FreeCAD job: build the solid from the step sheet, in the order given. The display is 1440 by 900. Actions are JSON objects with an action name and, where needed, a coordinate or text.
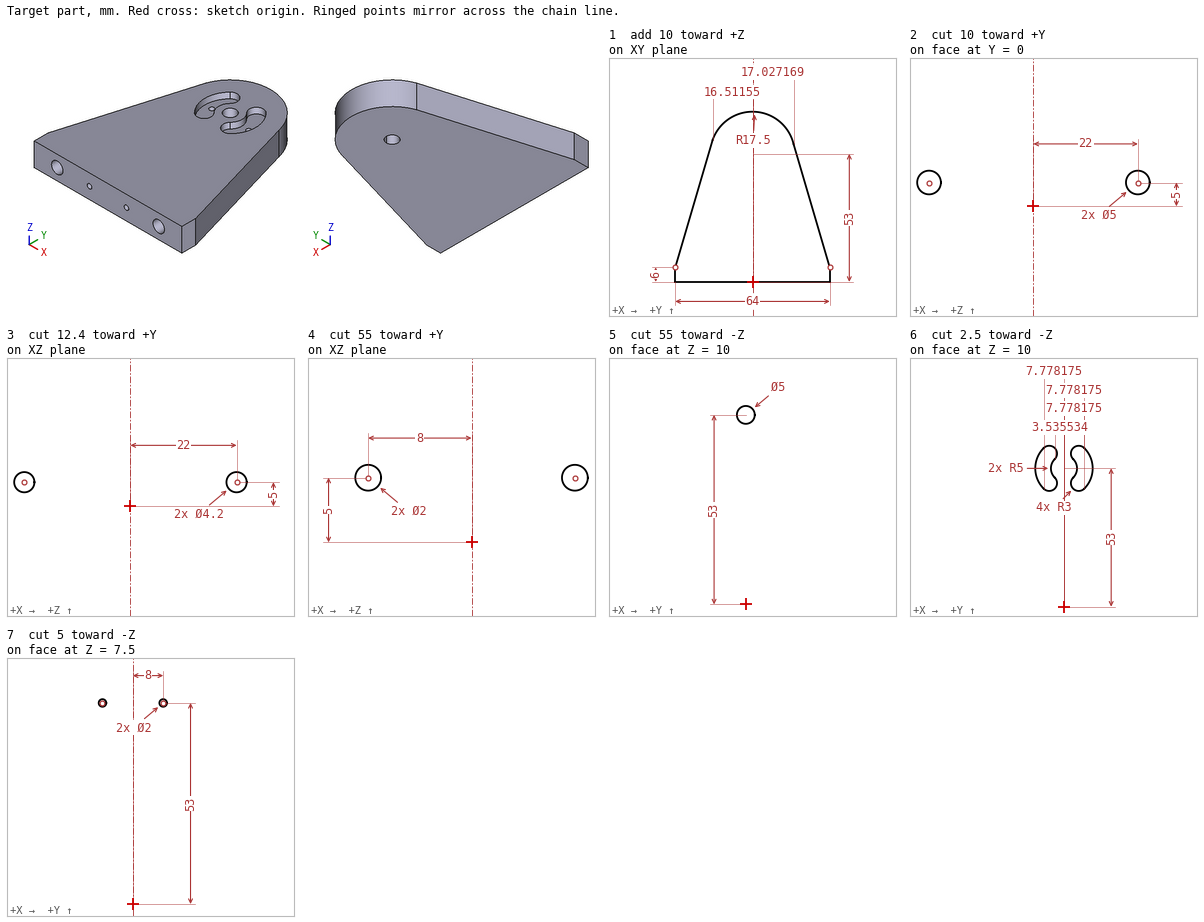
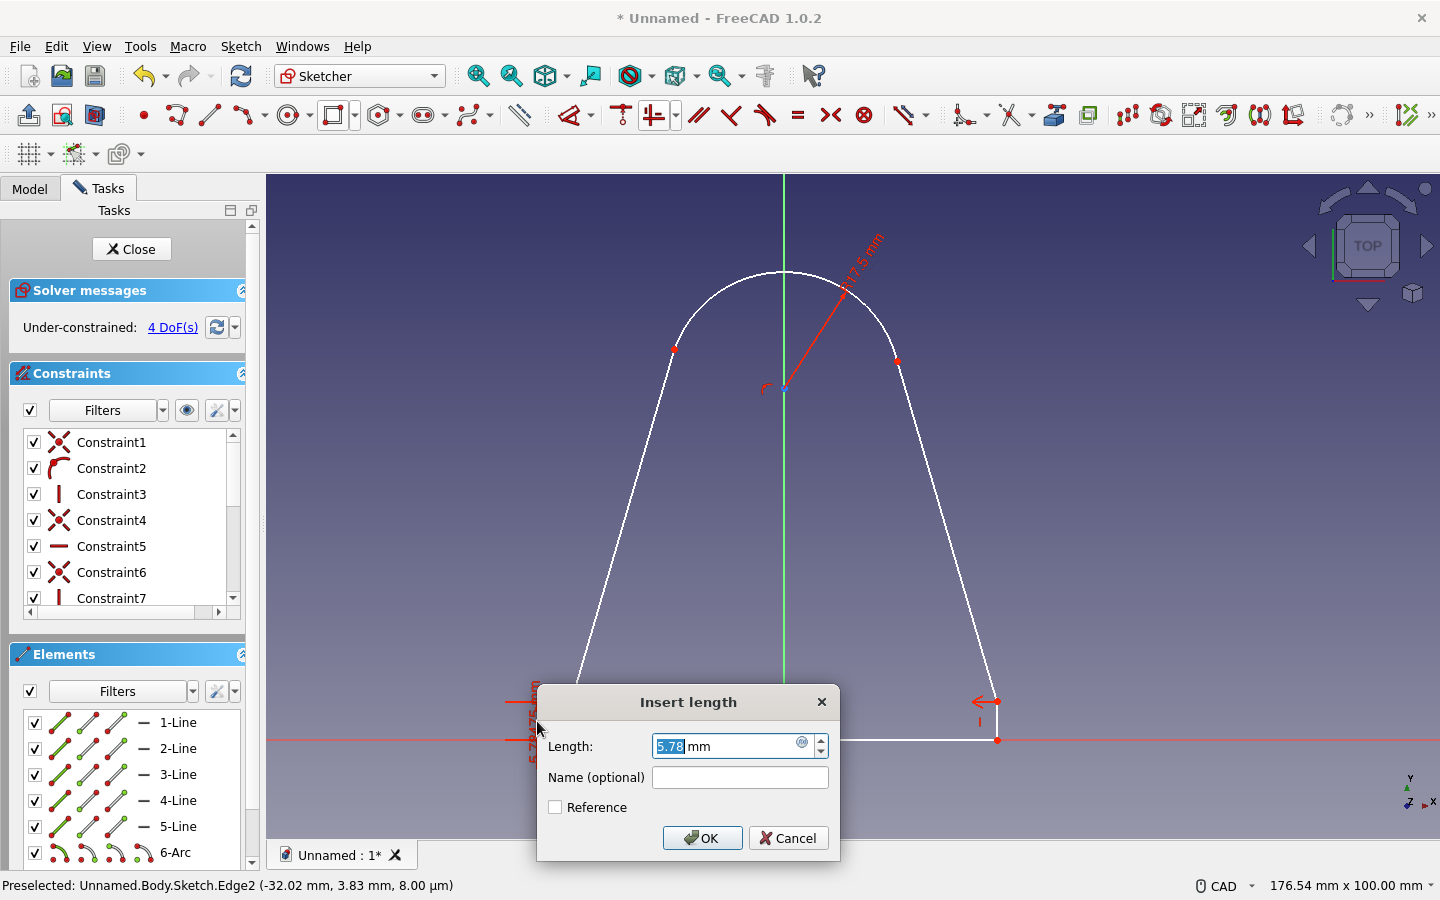
{"action": "type", "text": "6"}
{"action": "key", "text": "Return"}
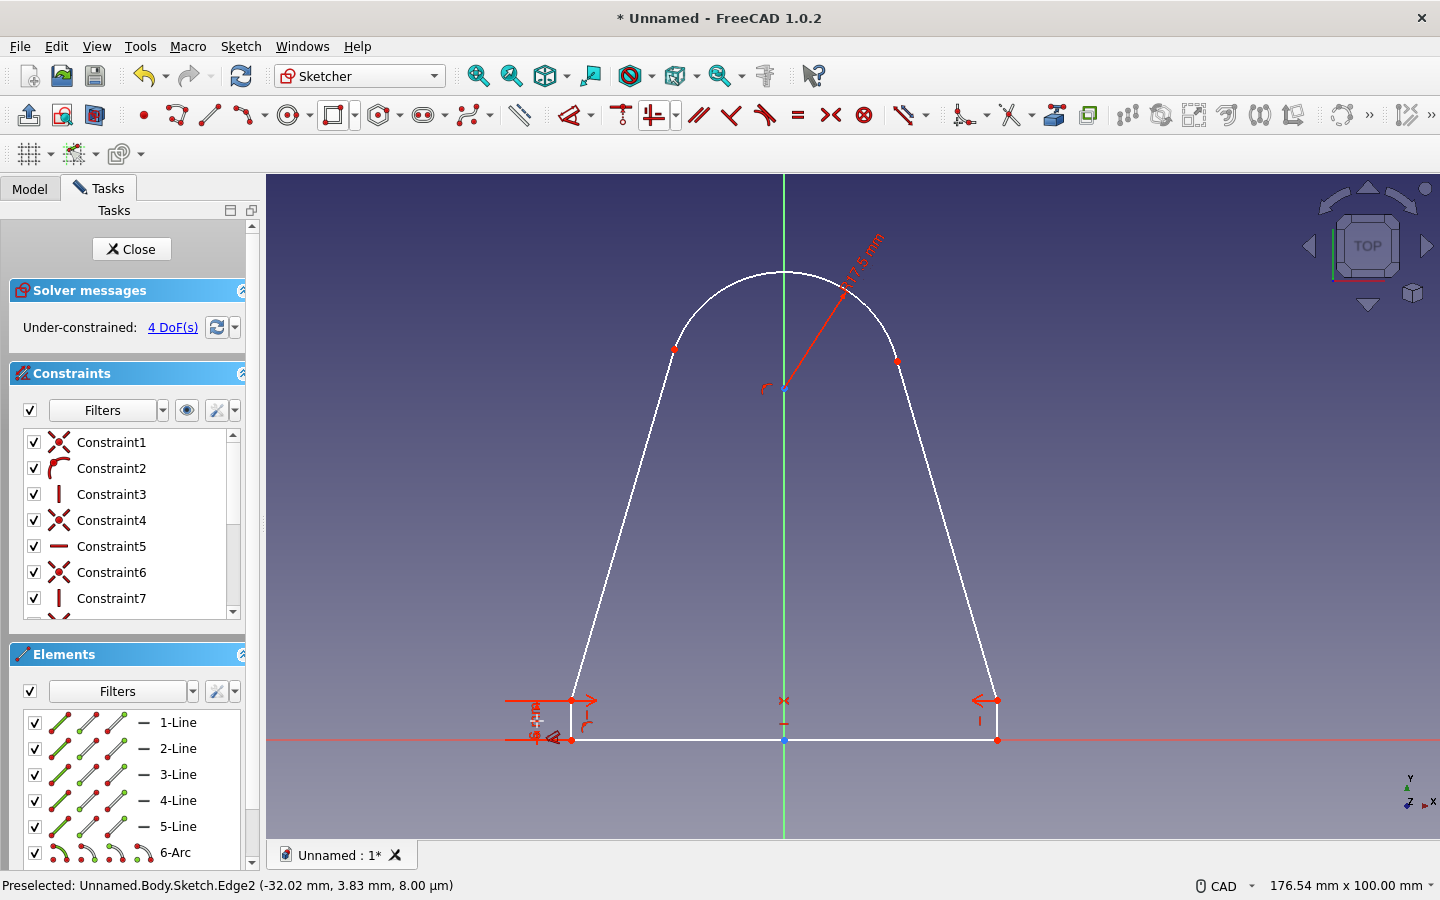
{"action": "left_click", "coordinate": [699, 740]}
{"action": "left_click", "coordinate": [686, 774]}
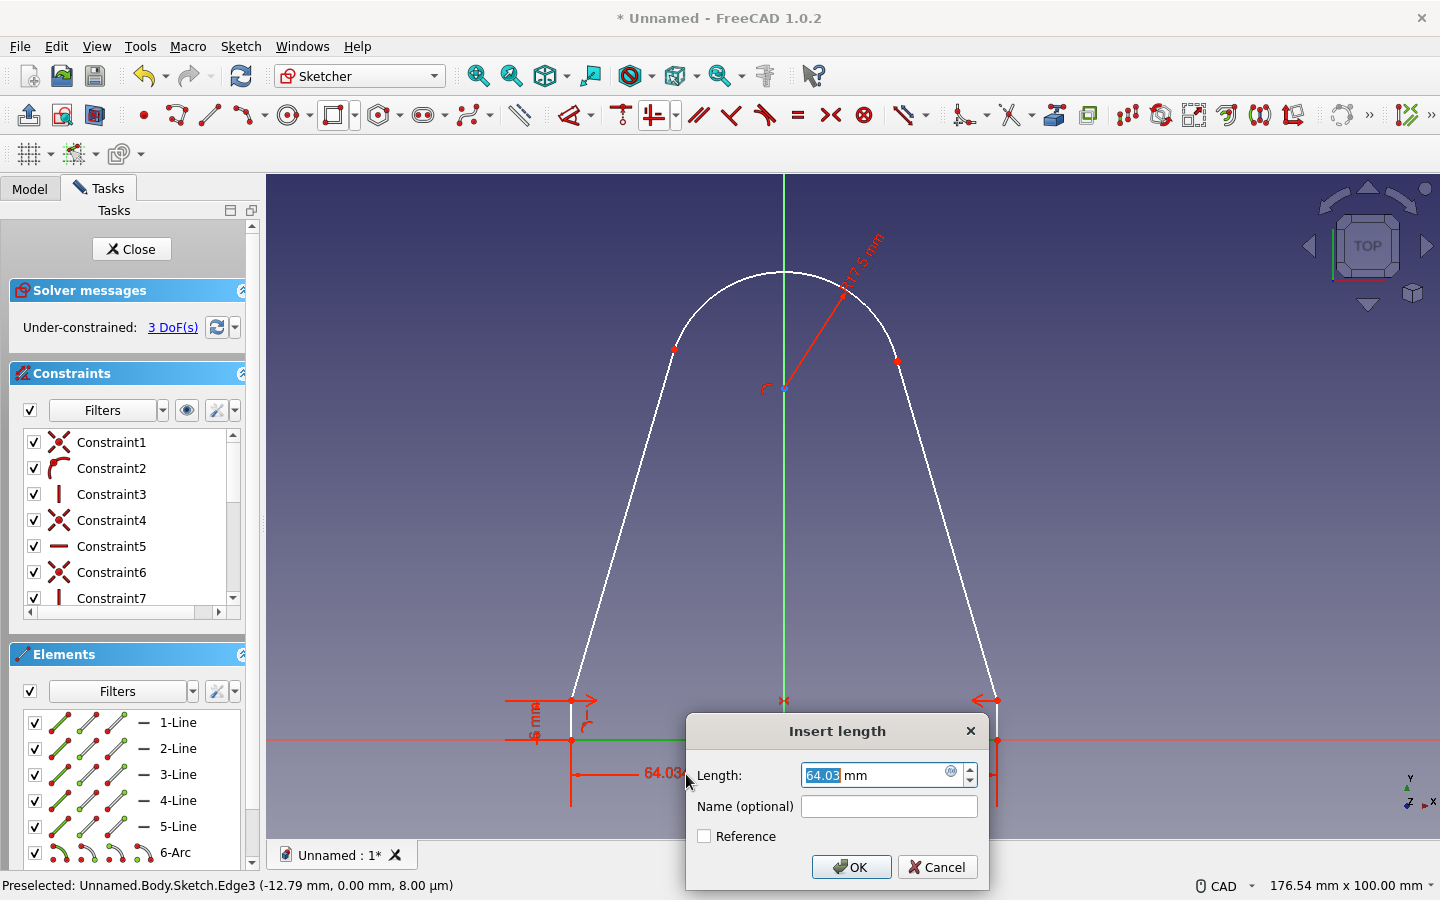
{"action": "type", "text": "64"}
{"action": "key", "text": "Return"}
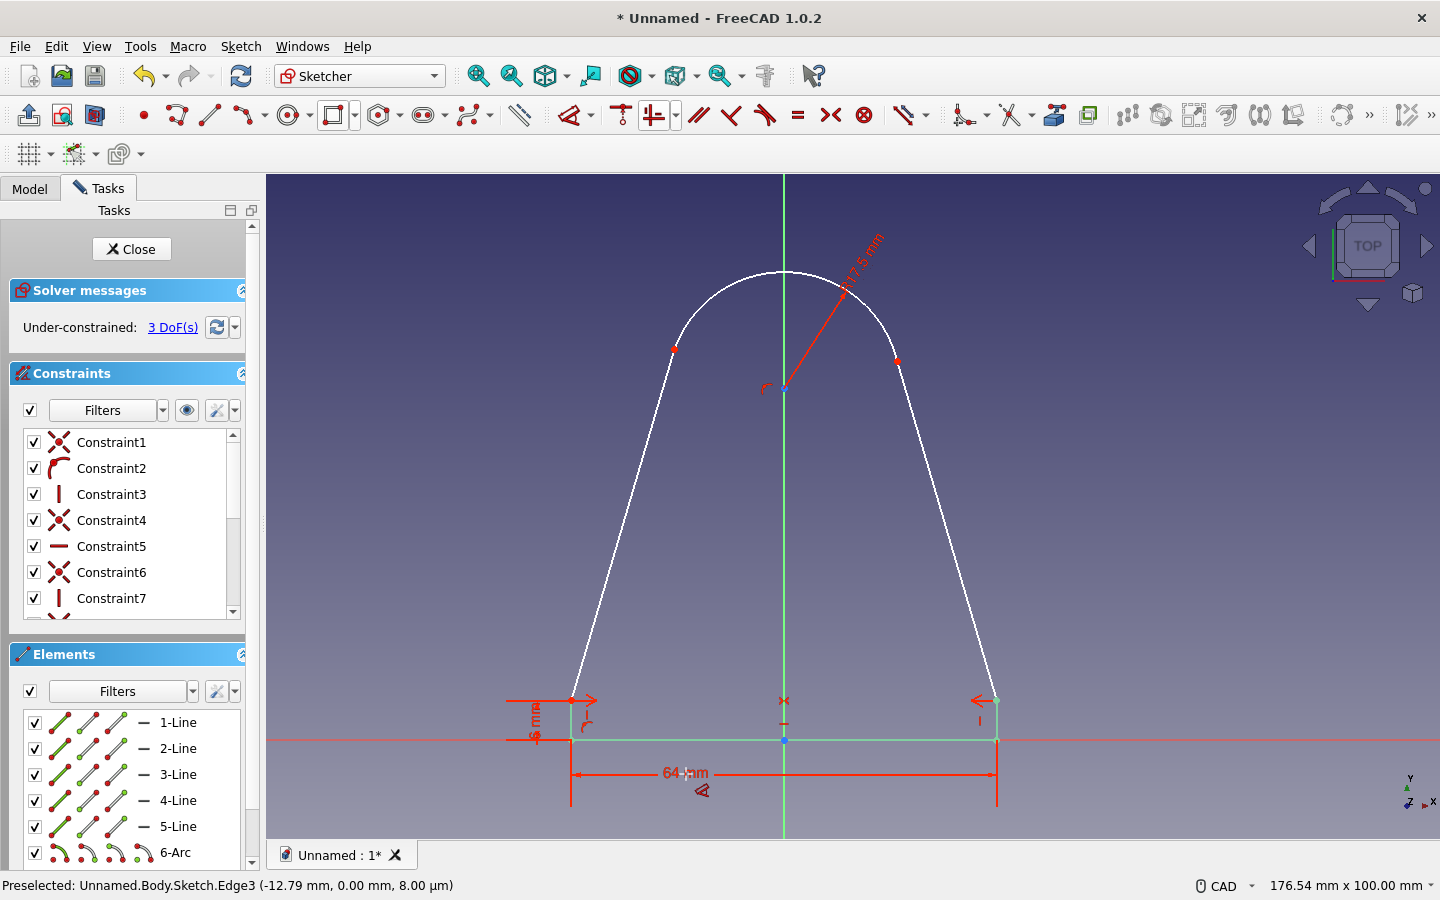
{"action": "left_click", "coordinate": [784, 389]}
{"action": "left_click", "coordinate": [818, 564]}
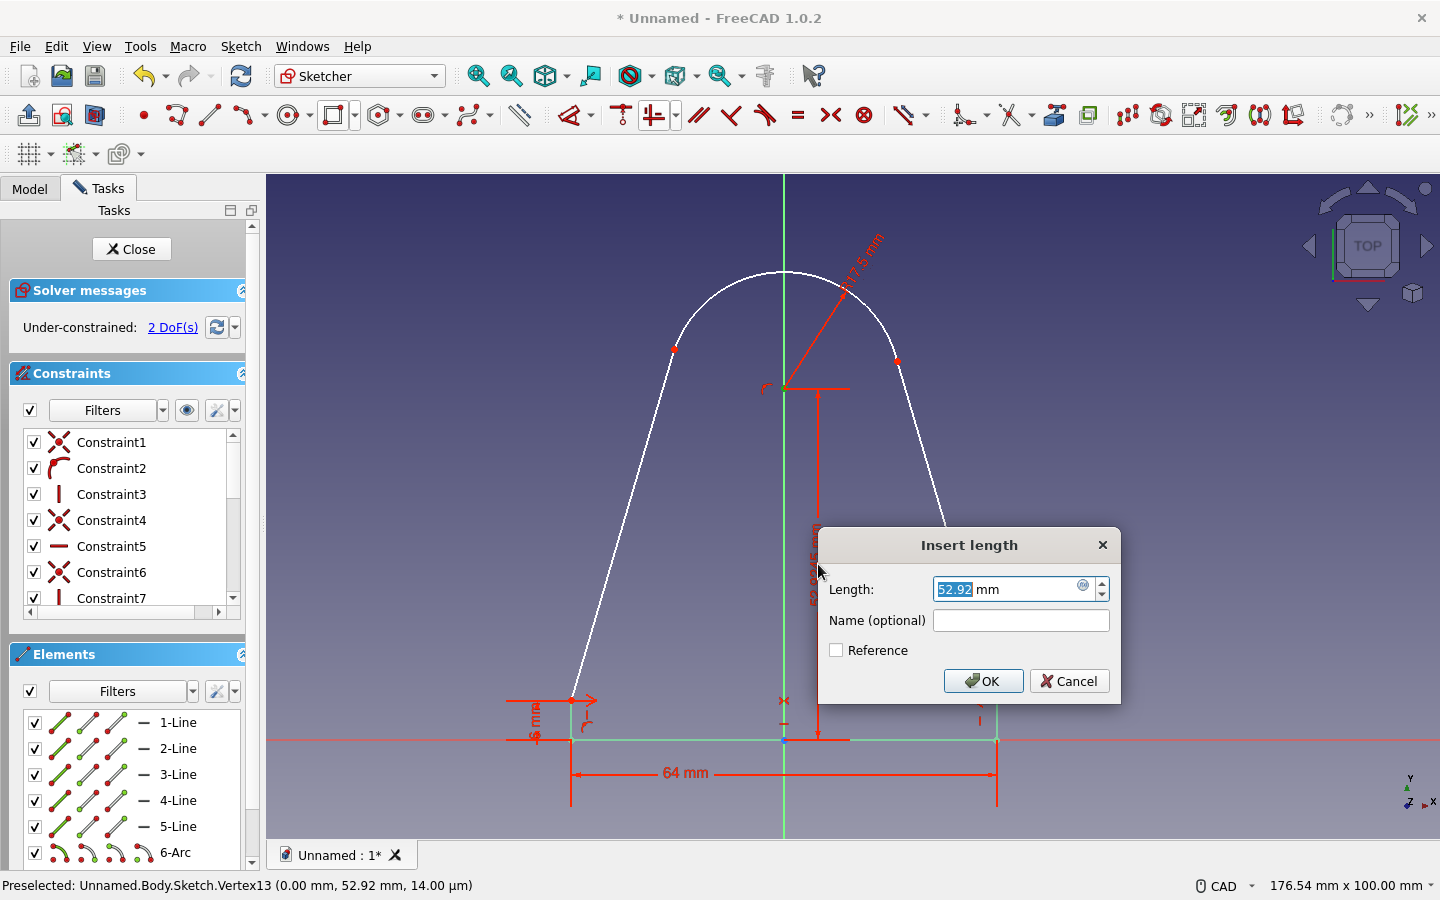
{"action": "type", "text": "53"}
{"action": "key", "text": "Return"}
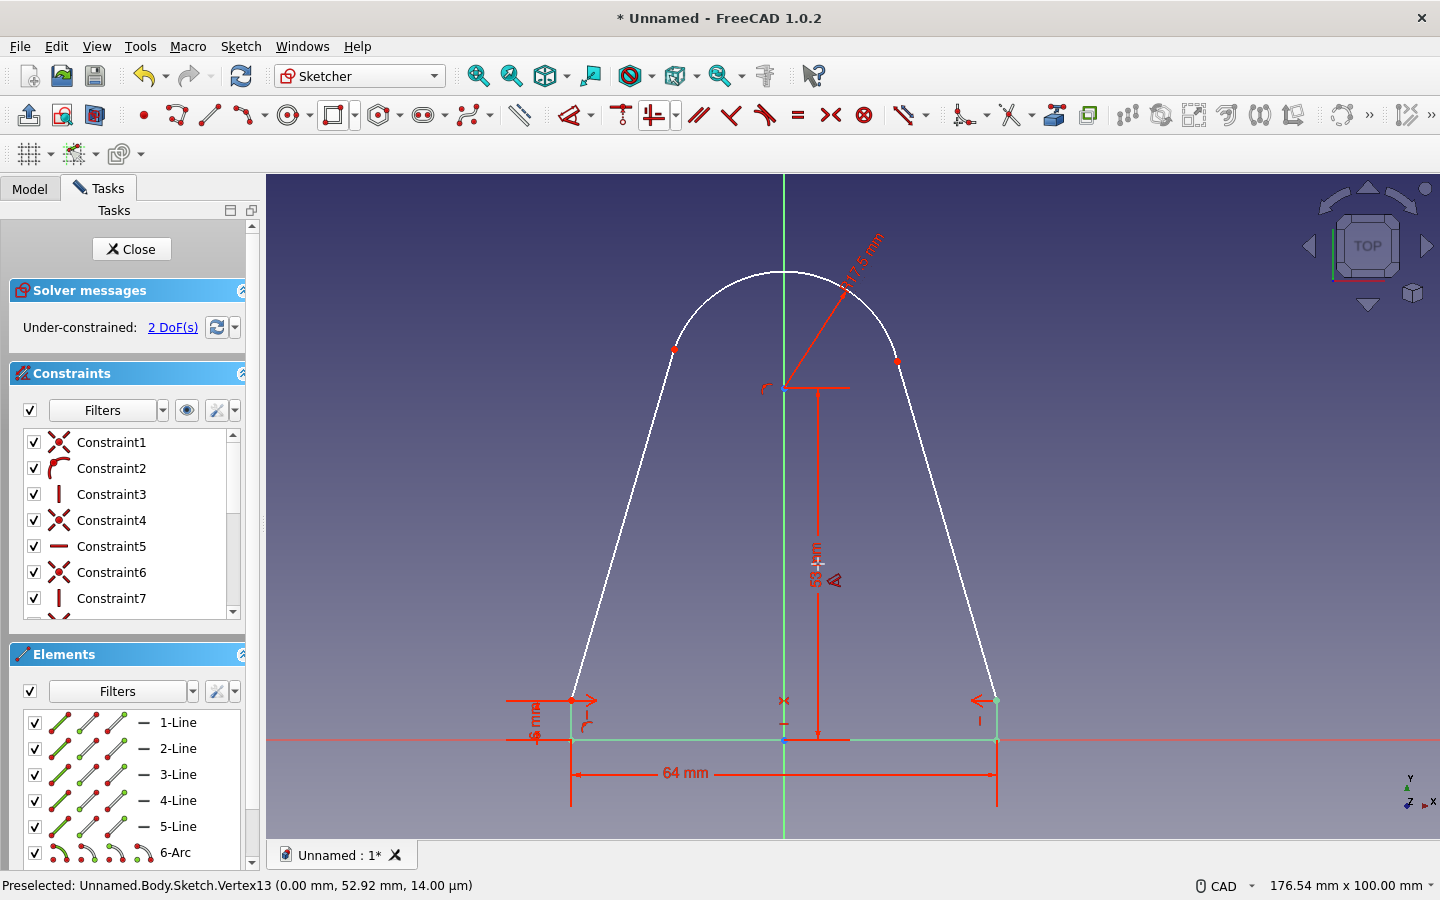
{"action": "left_click", "coordinate": [674, 350]}
{"action": "left_click", "coordinate": [768, 774]}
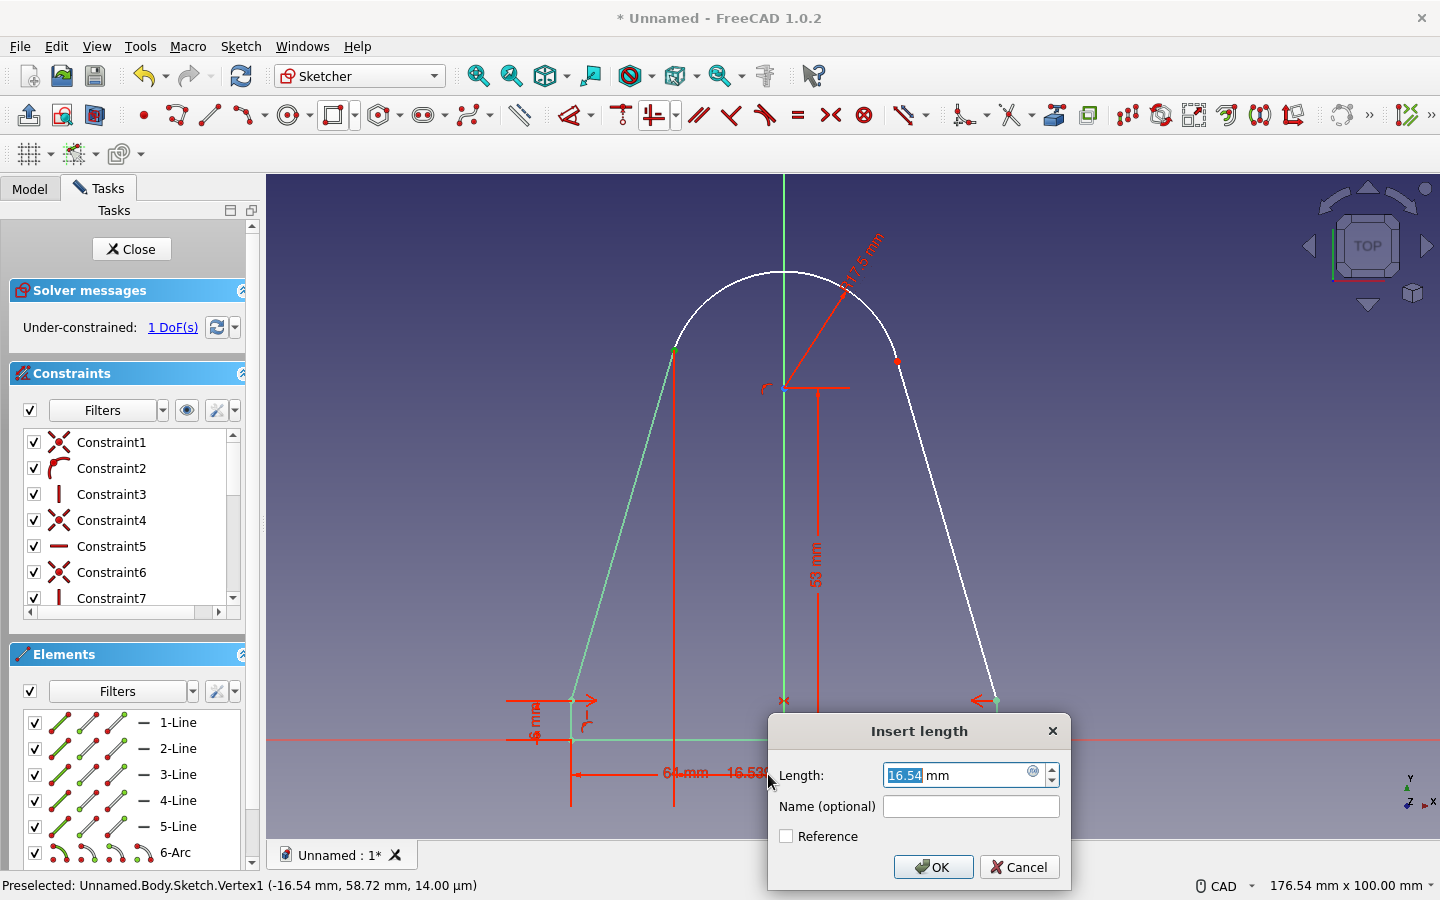
{"action": "type", "text": "16.51155"}
{"action": "key", "text": "Return"}